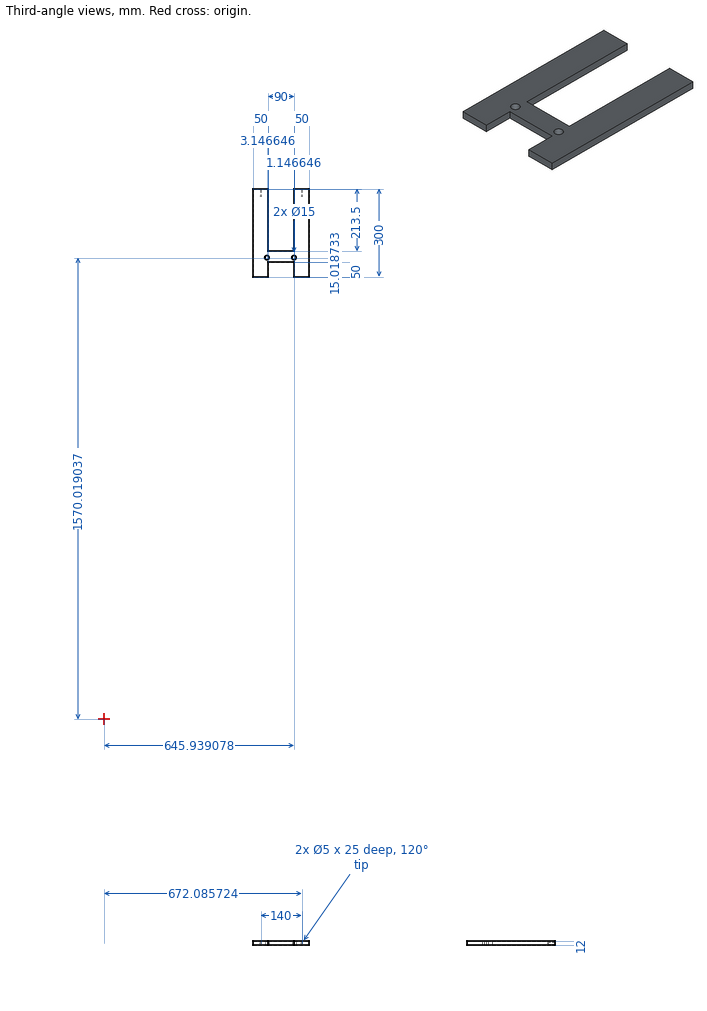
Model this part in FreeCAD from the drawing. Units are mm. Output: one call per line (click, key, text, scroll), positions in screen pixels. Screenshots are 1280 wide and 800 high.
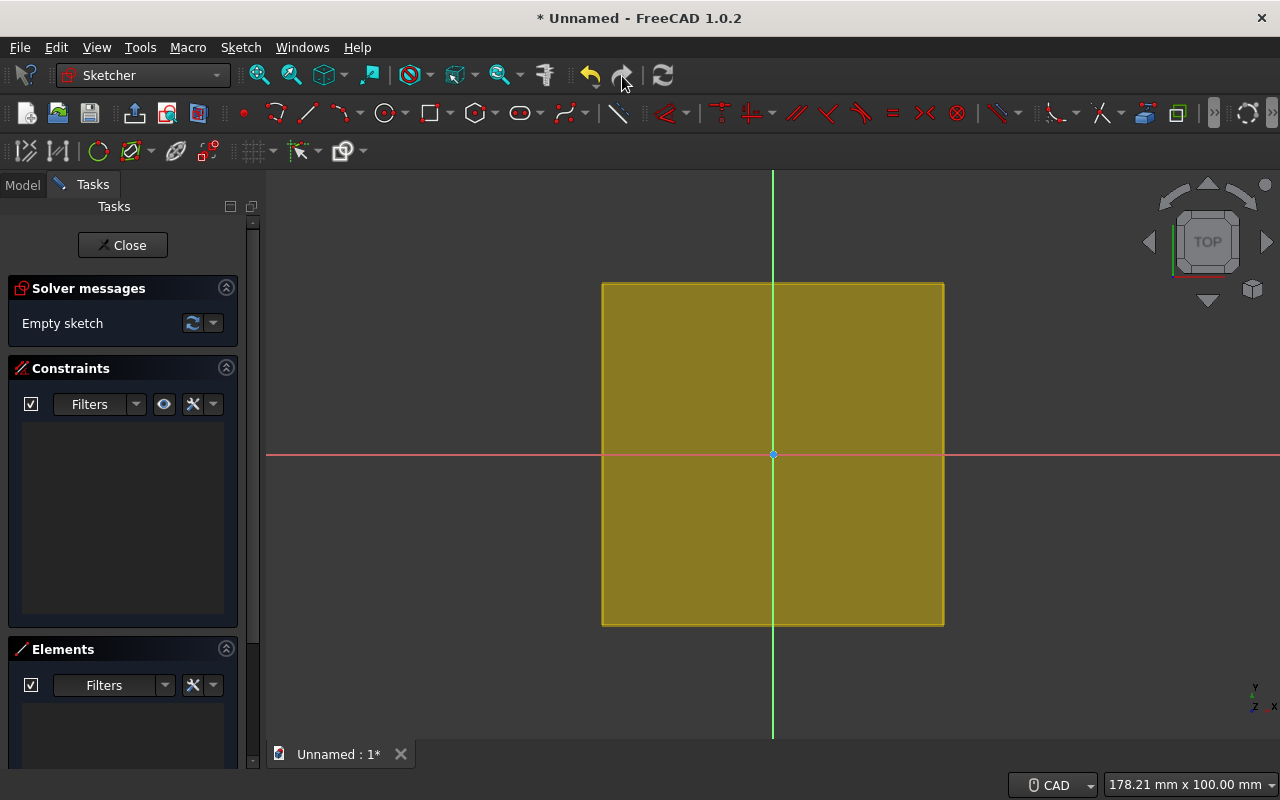
scroll(704, 454, down, 8)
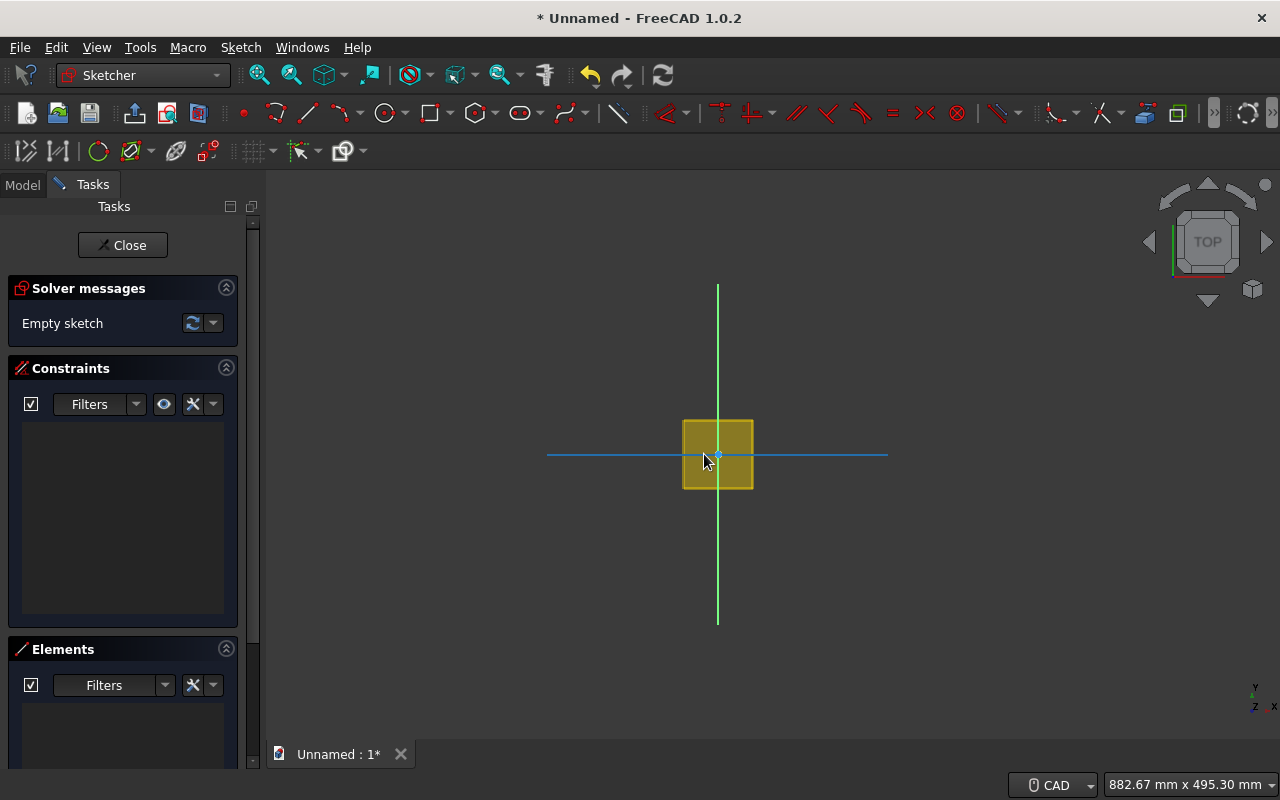
scroll(704, 454, down, 5)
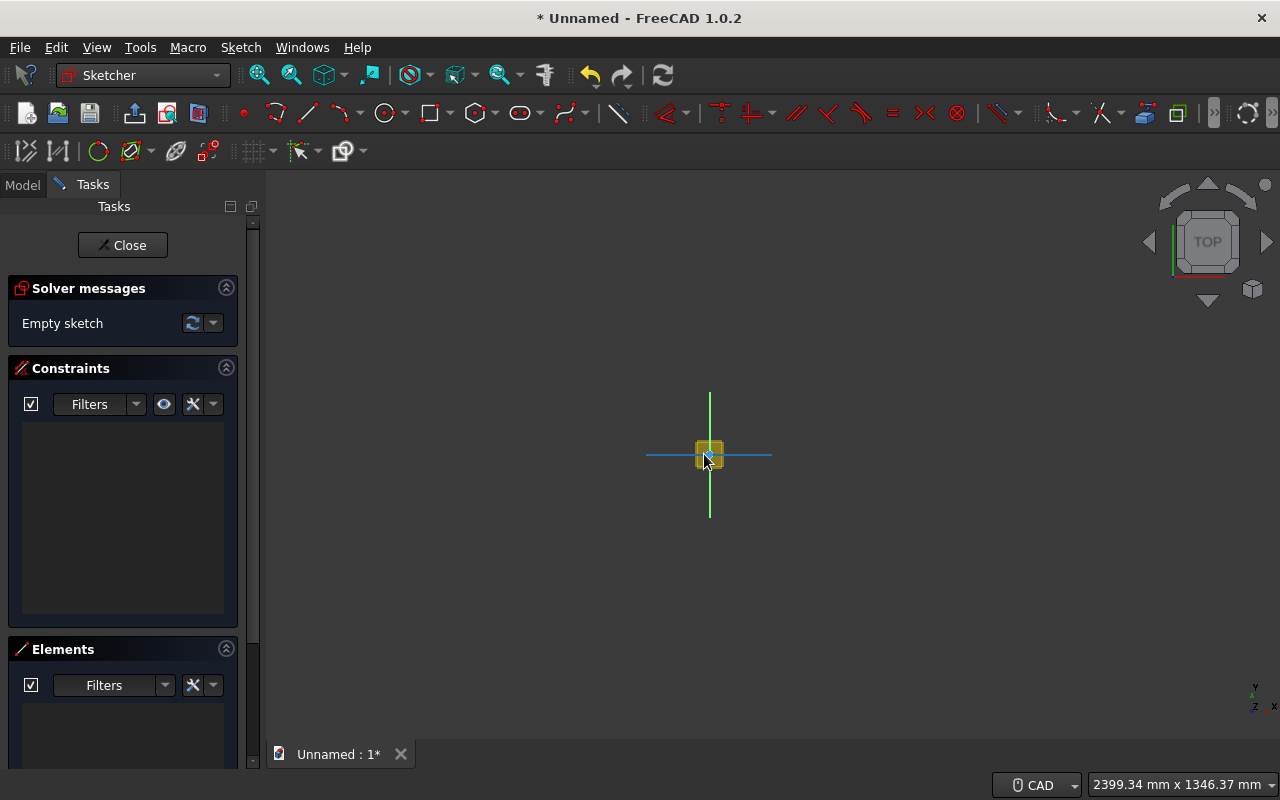
scroll(704, 454, down, 5)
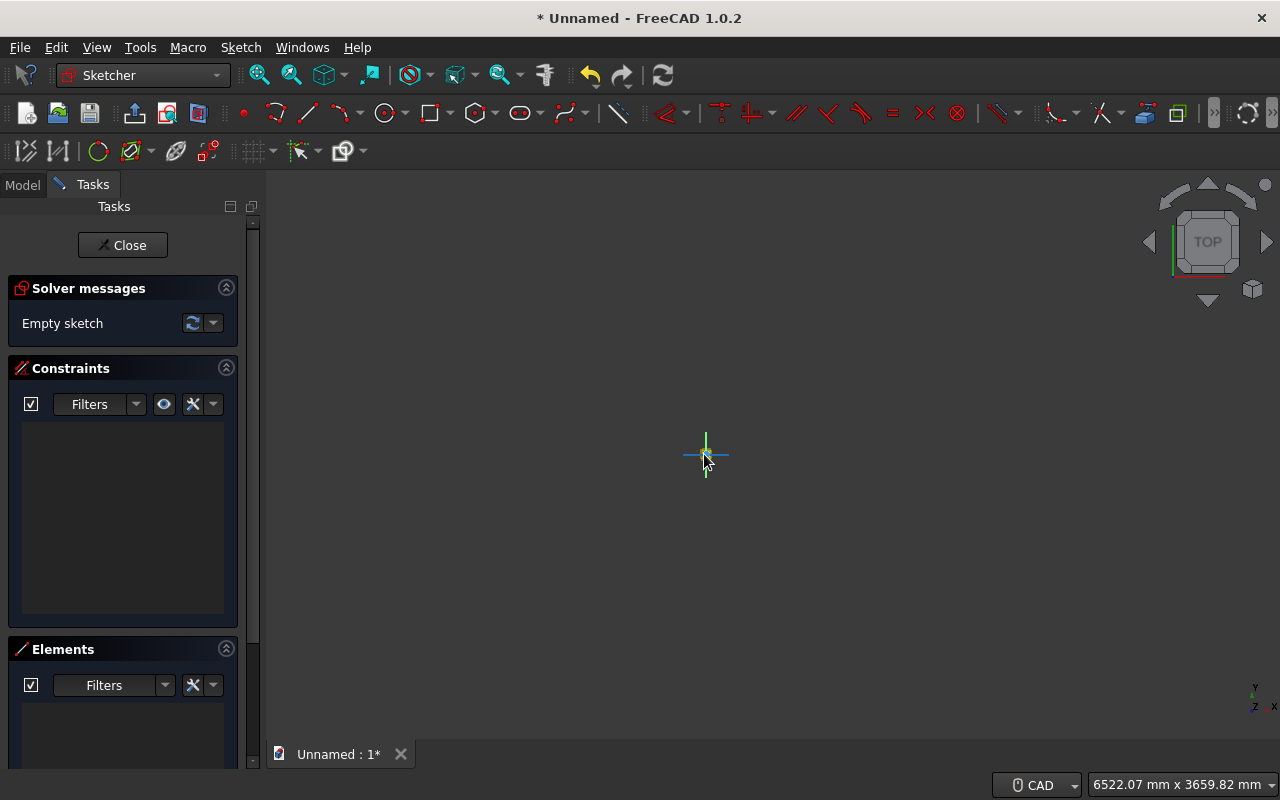
scroll(704, 454, down, 5)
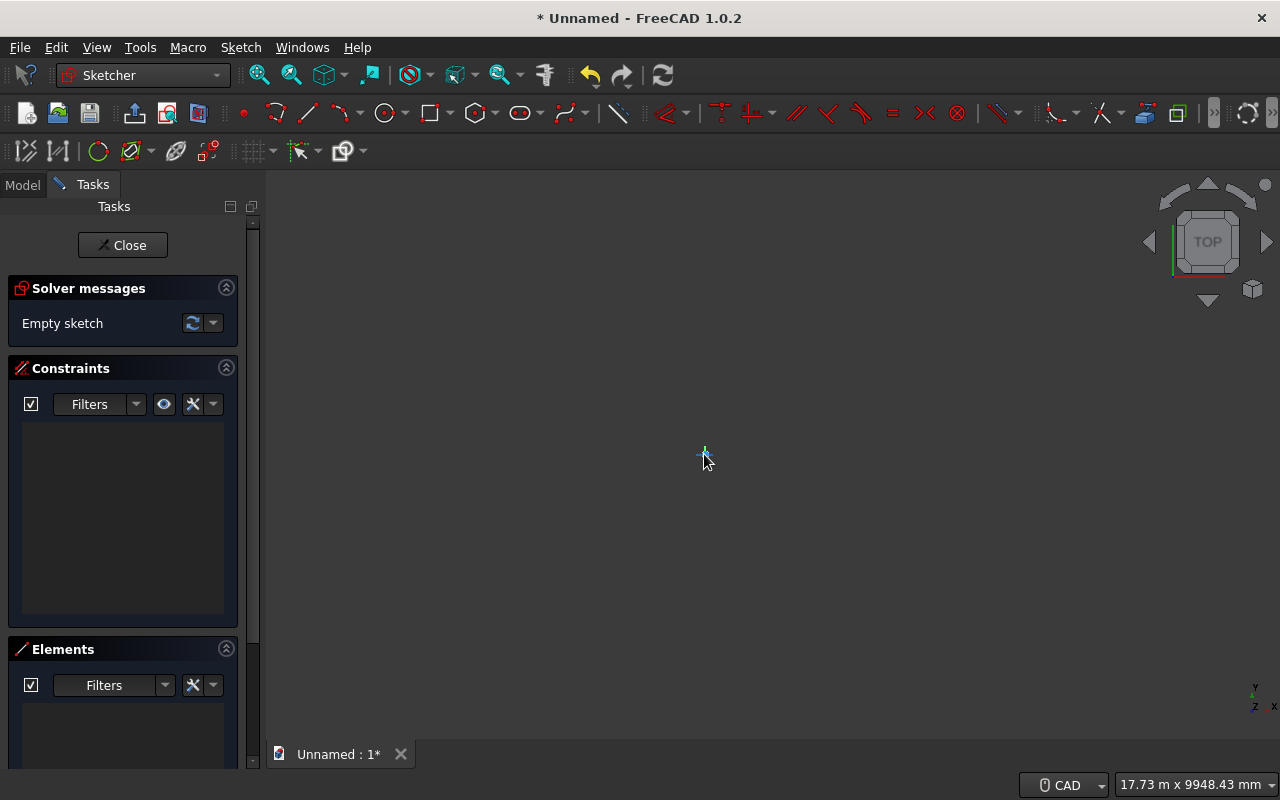
scroll(741, 355, up, 15)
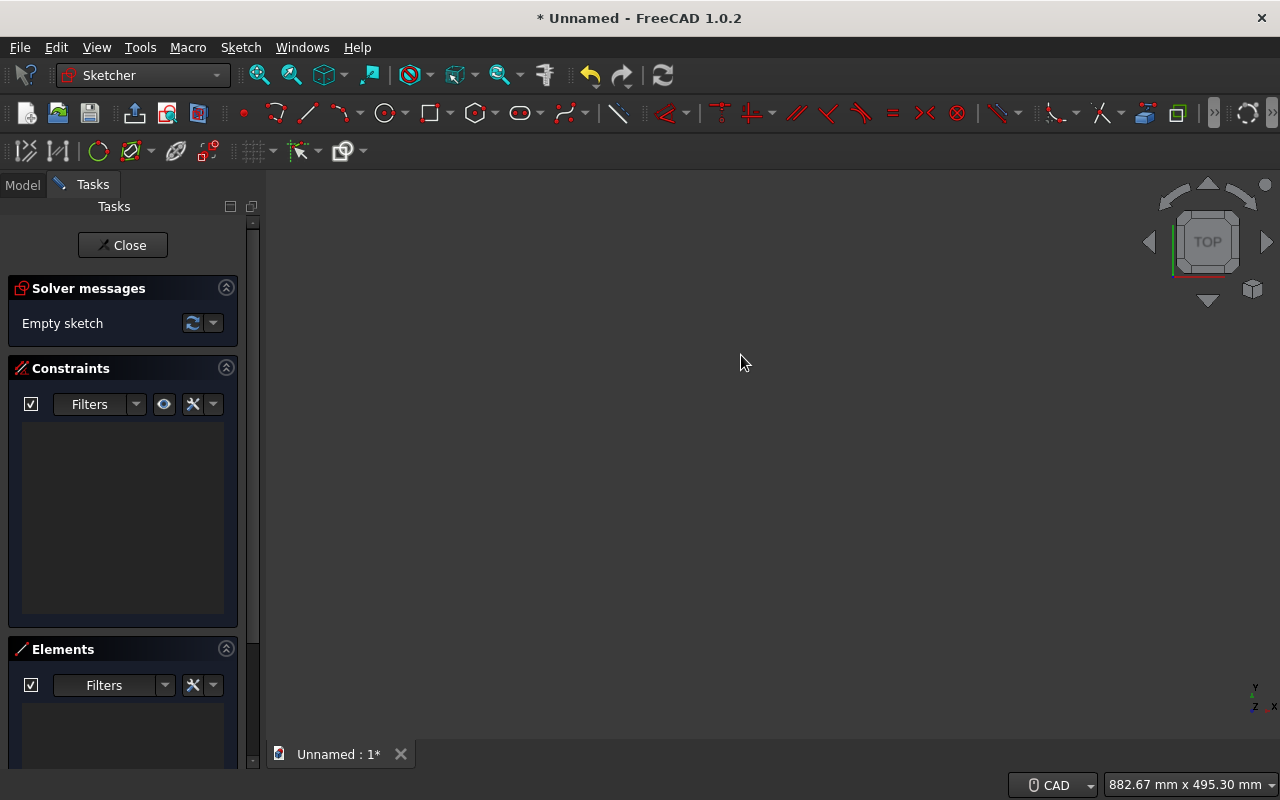
key(g)
key(m)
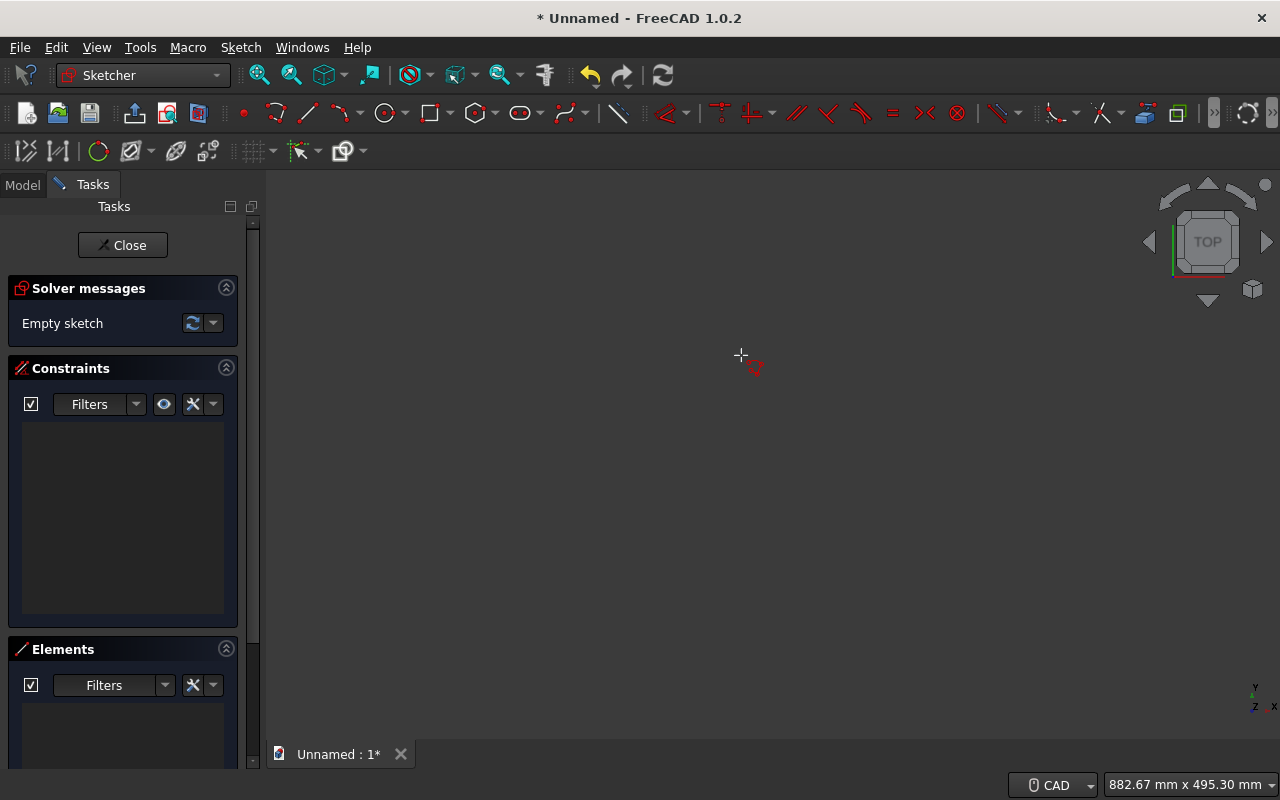
click(594, 618)
click(594, 274)
click(651, 274)
click(651, 519)
click(755, 519)
click(755, 274)
click(812, 274)
click(812, 618)
click(755, 618)
click(755, 561)
click(651, 561)
click(651, 618)
click(594, 619)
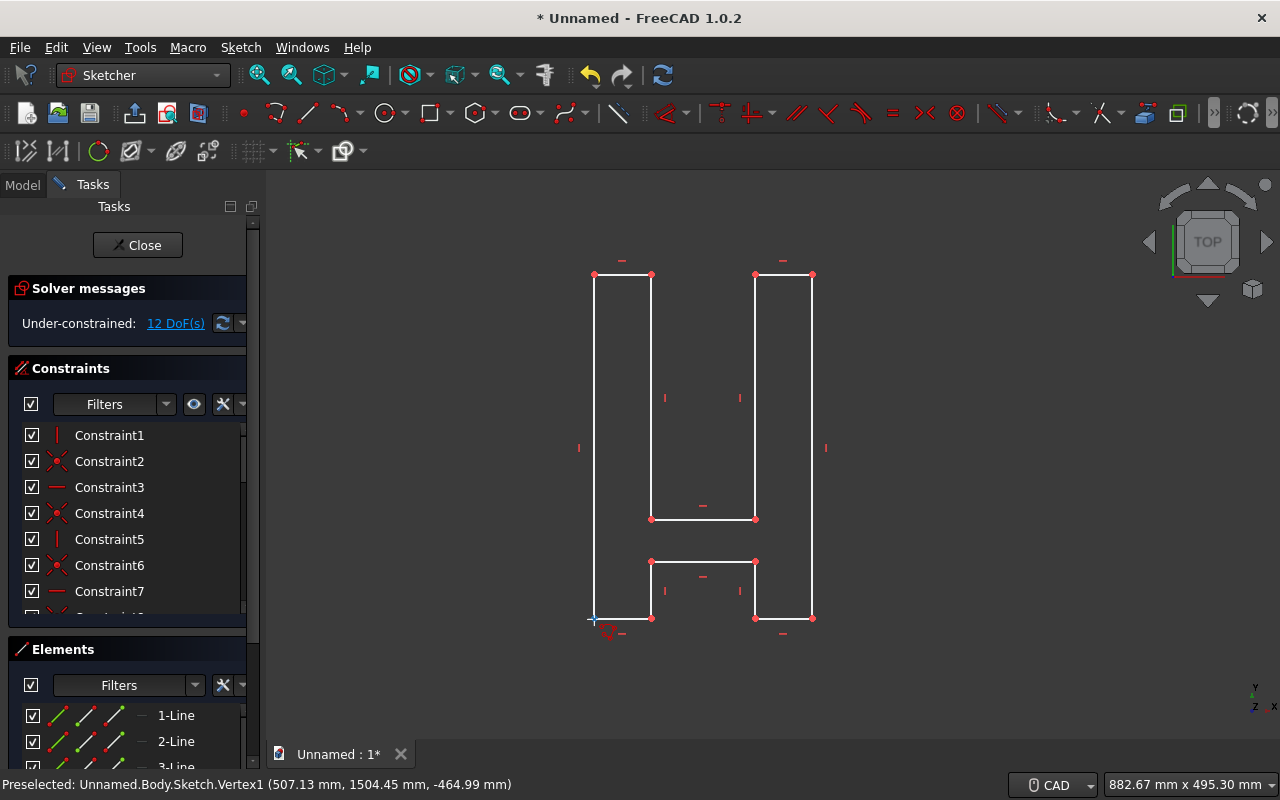
click(386, 114)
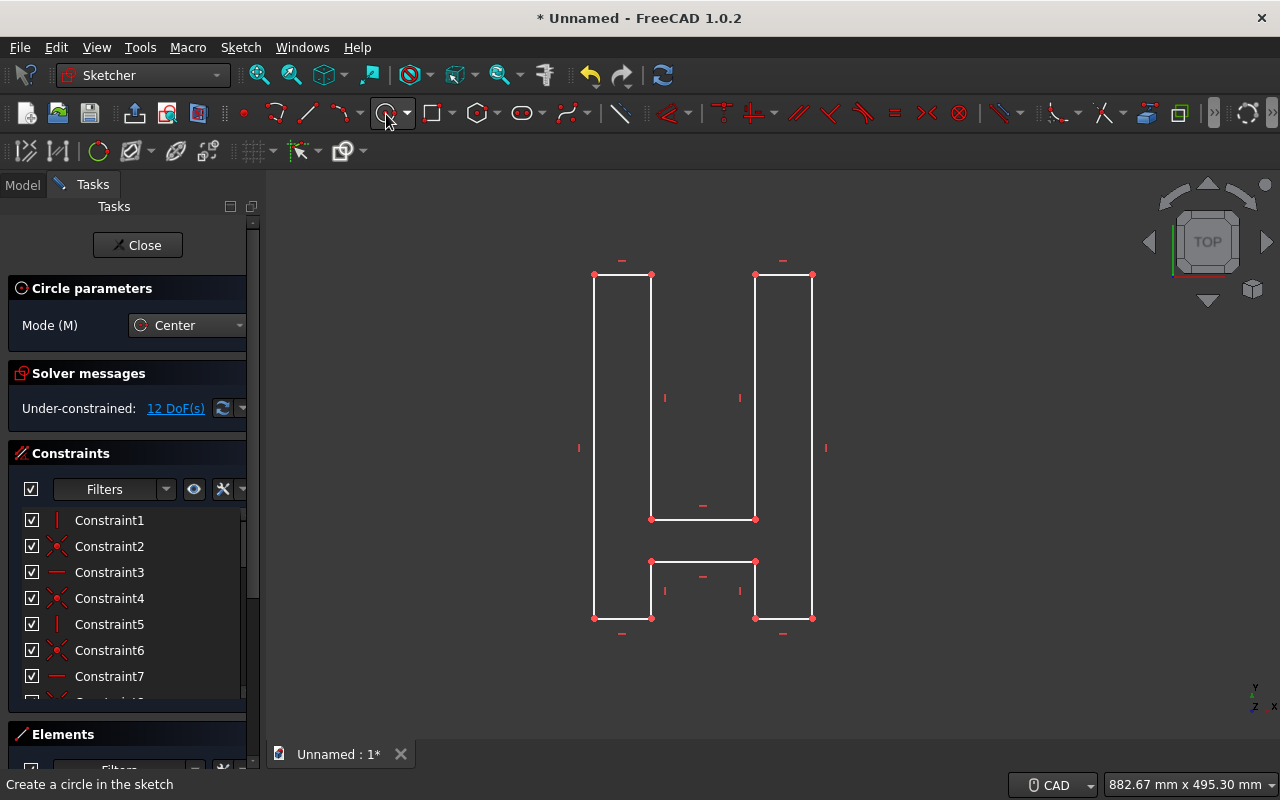
scroll(753, 544, up, 5)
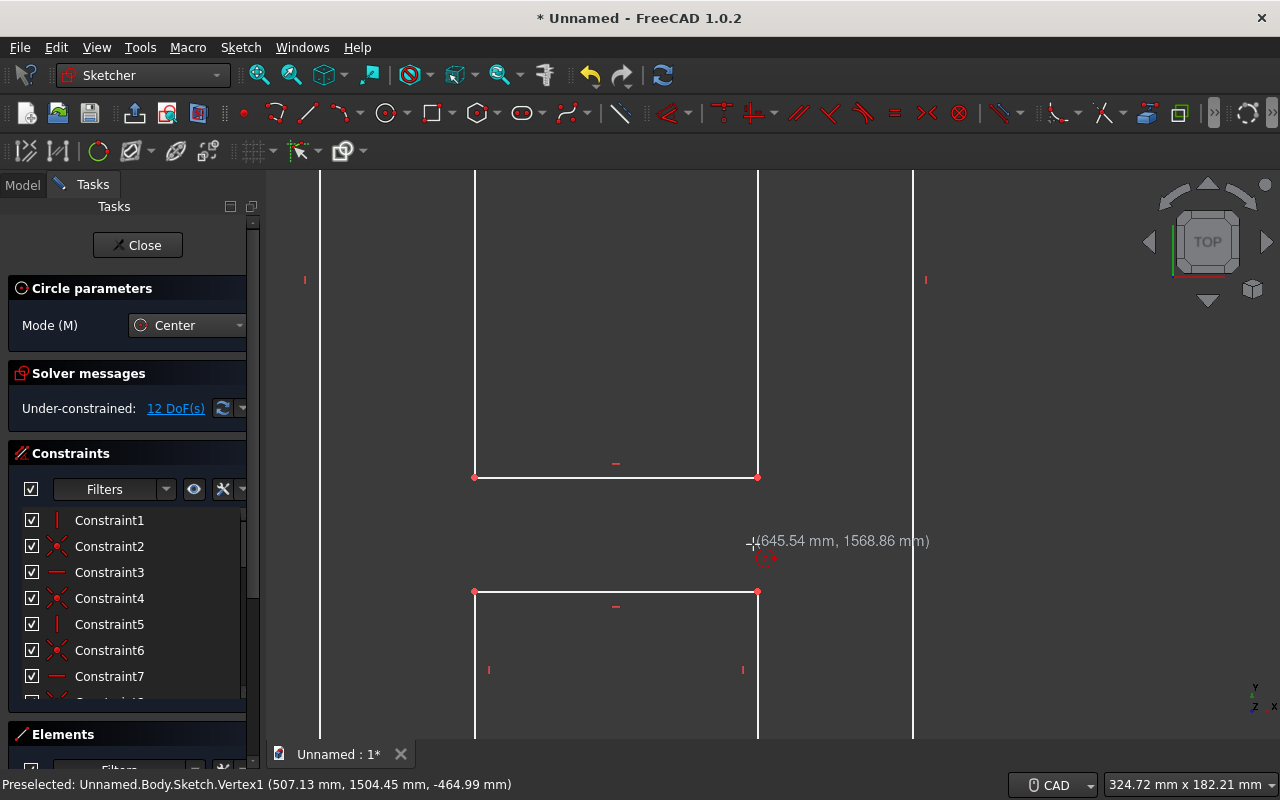
click(753, 542)
move(770, 525)